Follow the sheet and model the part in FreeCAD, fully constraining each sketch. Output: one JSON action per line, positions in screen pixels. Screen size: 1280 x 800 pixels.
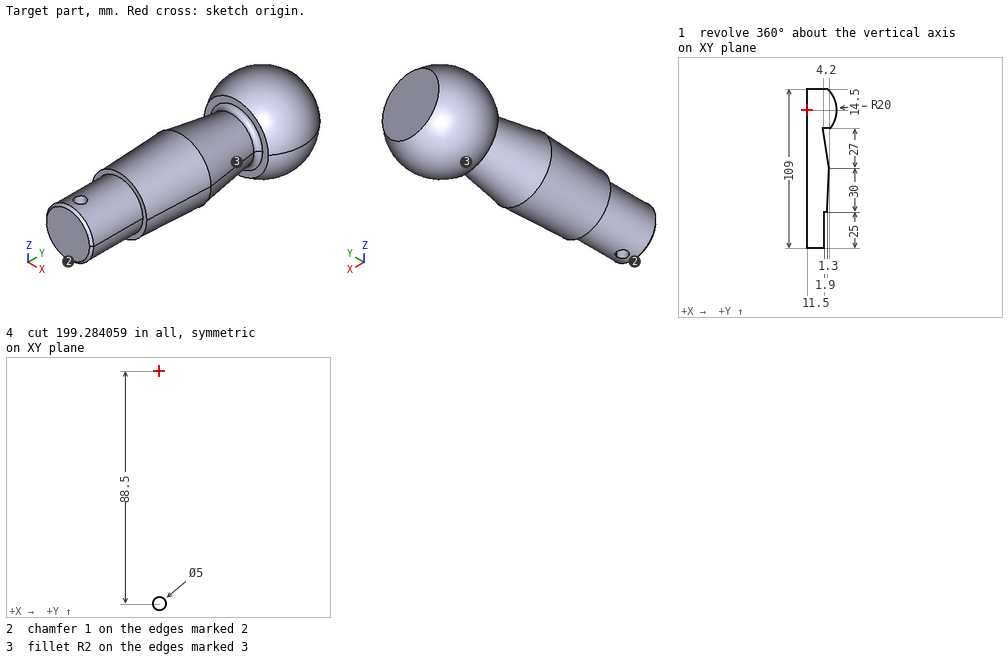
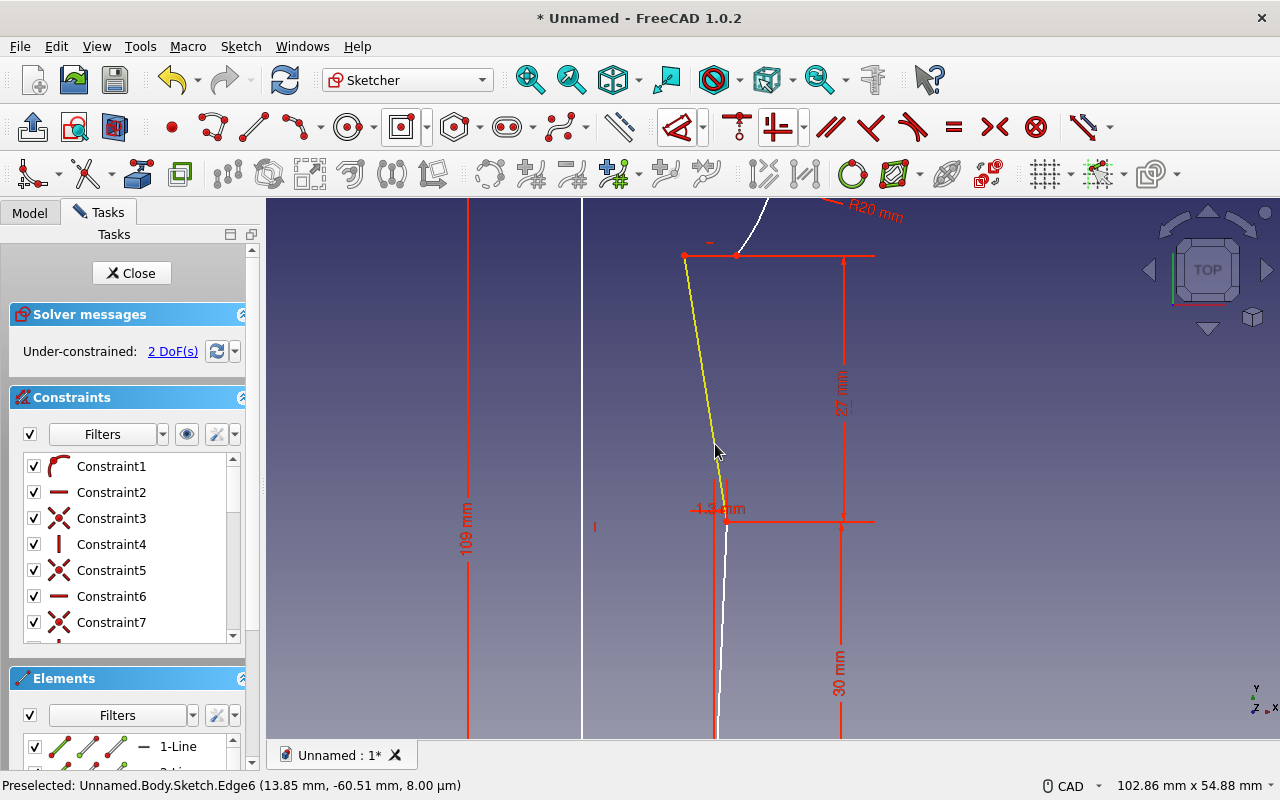
{"action": "left_click", "coordinate": [714, 442]}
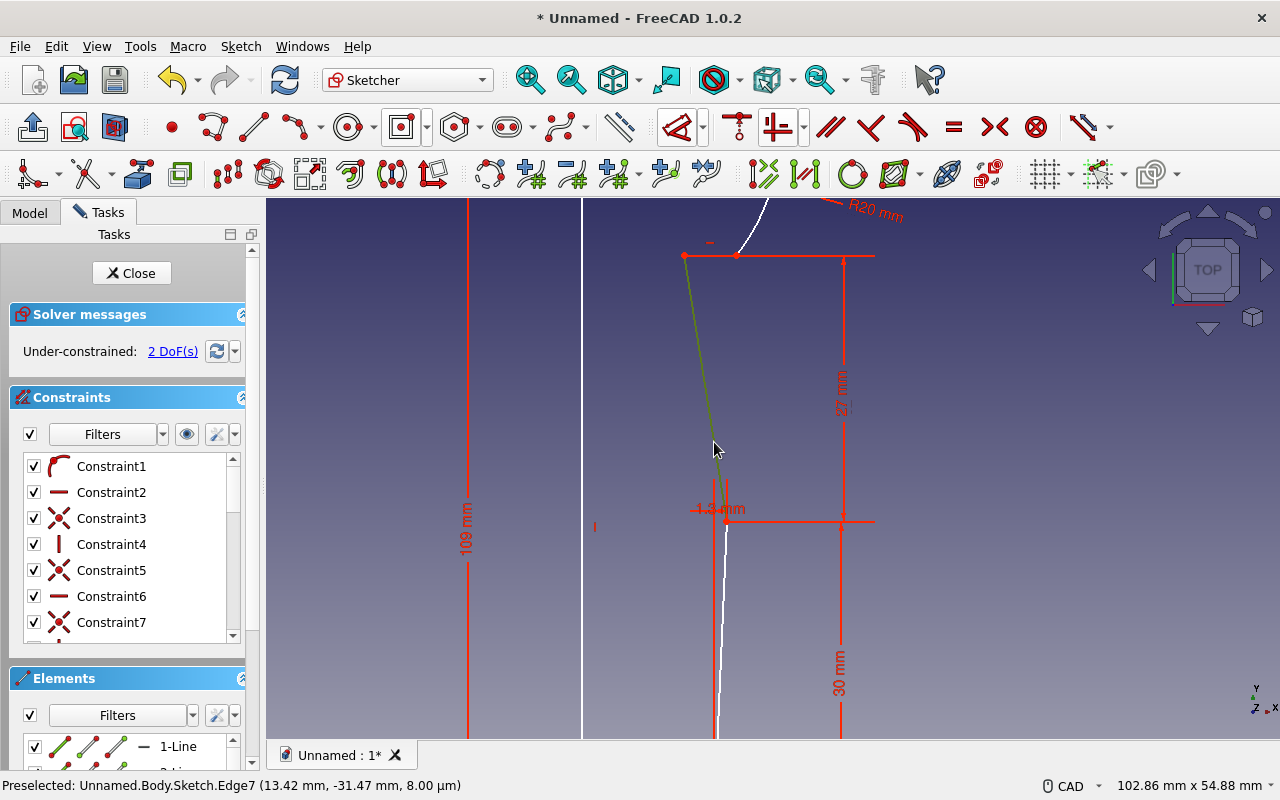
{"action": "left_click", "coordinate": [702, 128]}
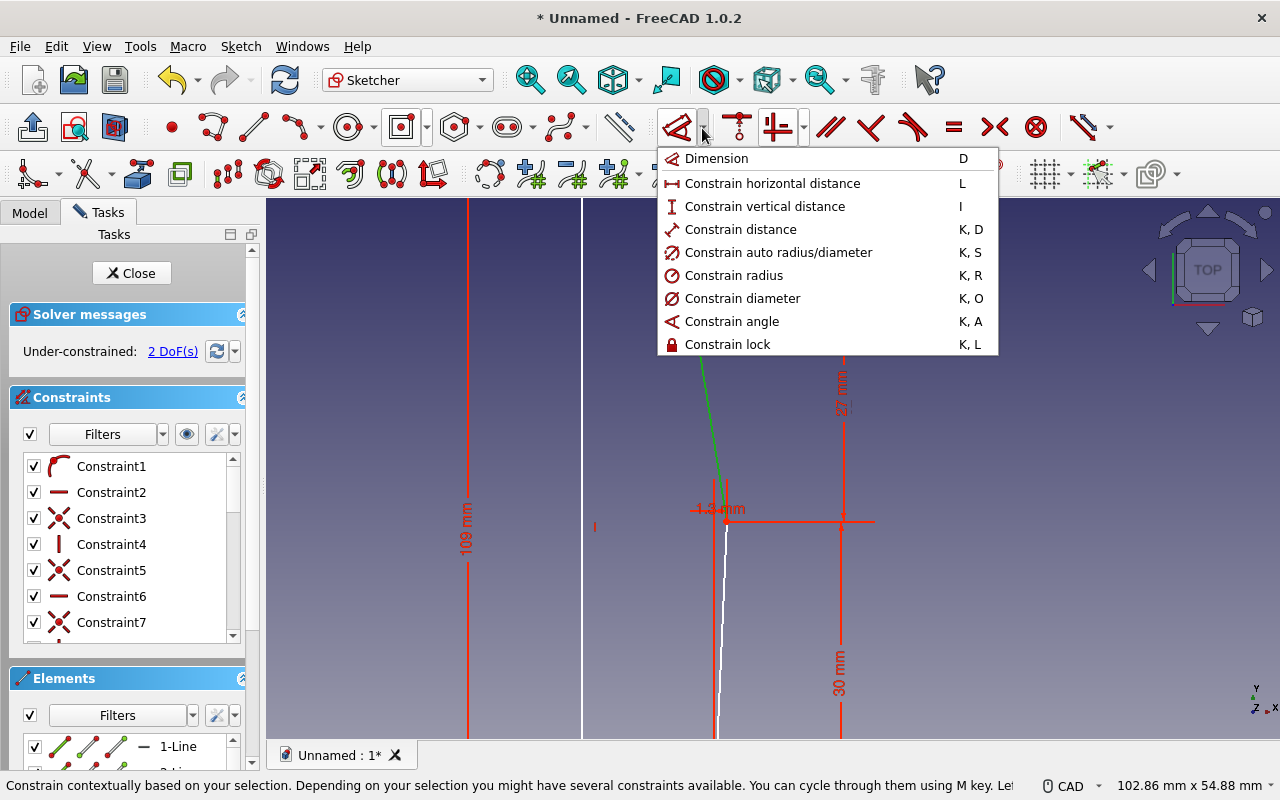
{"action": "left_click", "coordinate": [828, 184]}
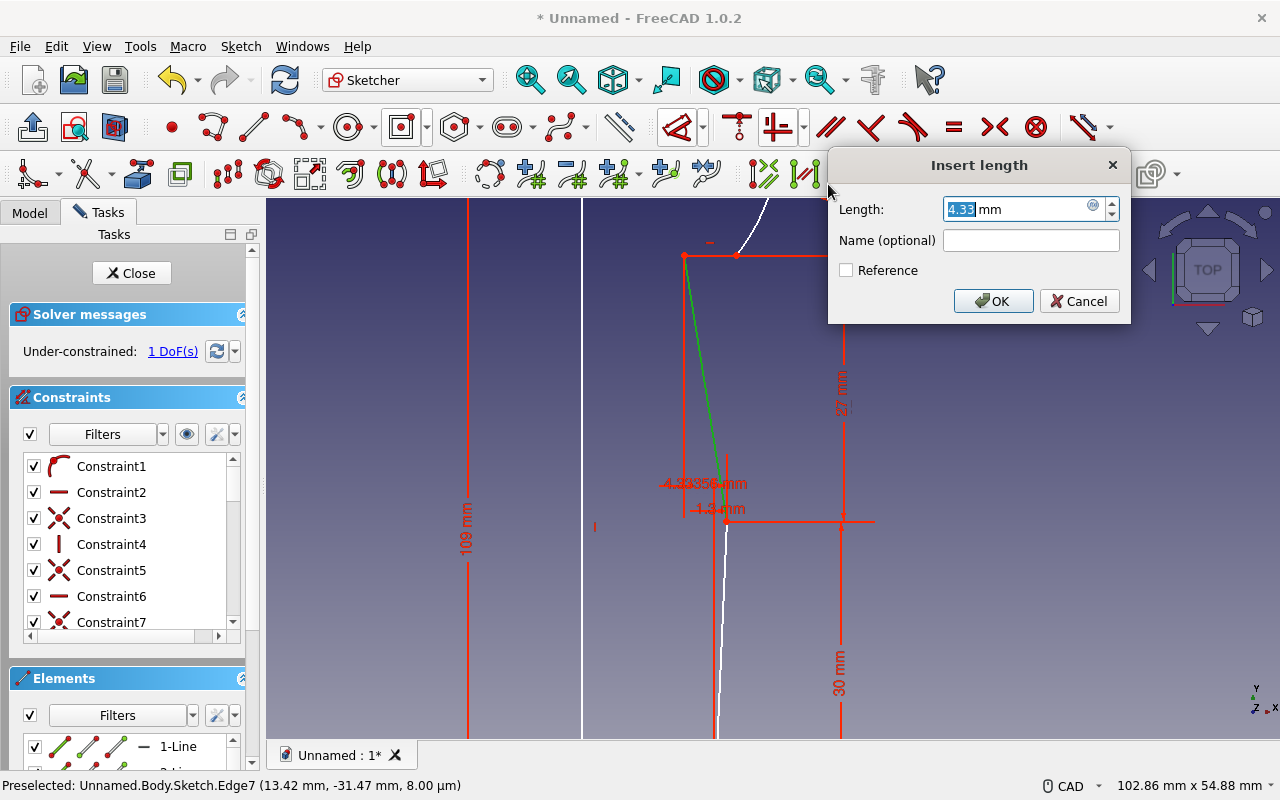
{"action": "type", "text": "4.2"}
{"action": "key", "text": "Return"}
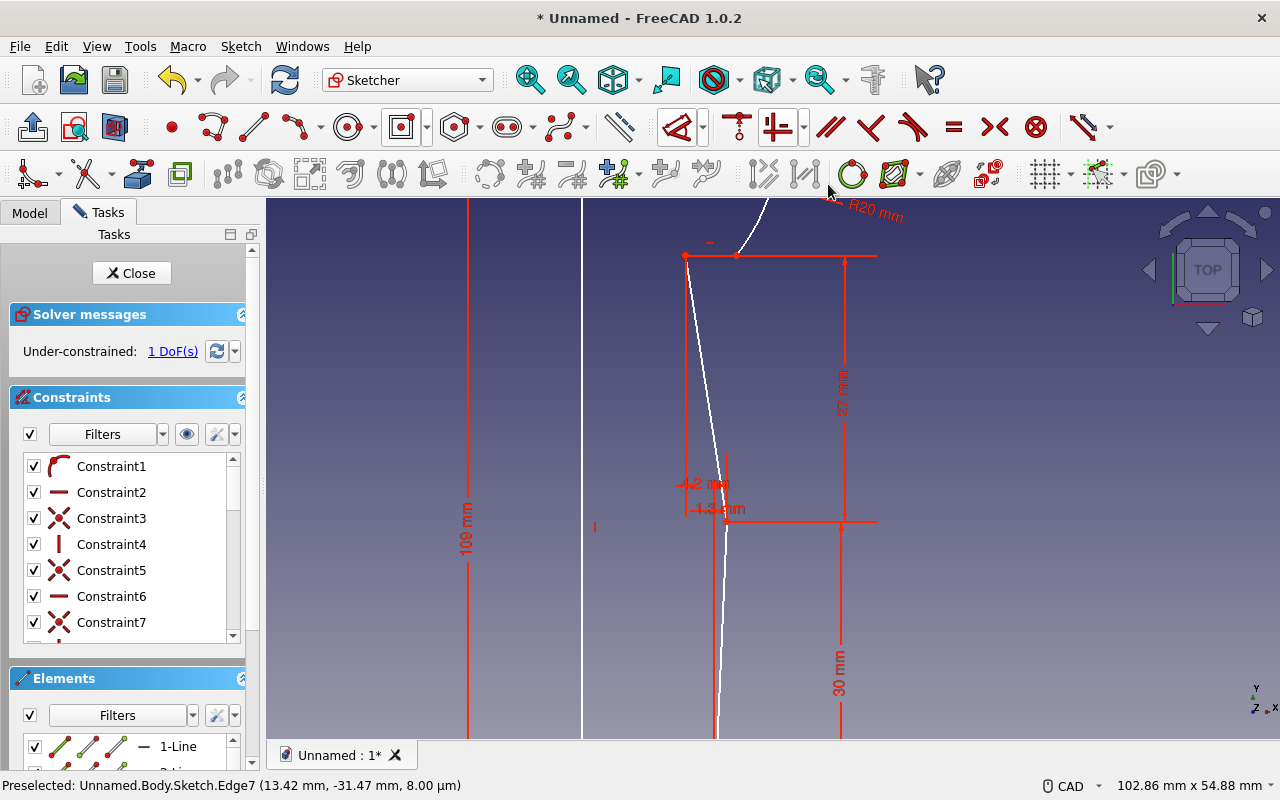
{"action": "scroll", "coordinate": [715, 443], "scroll_direction": "down", "scroll_amount": 6}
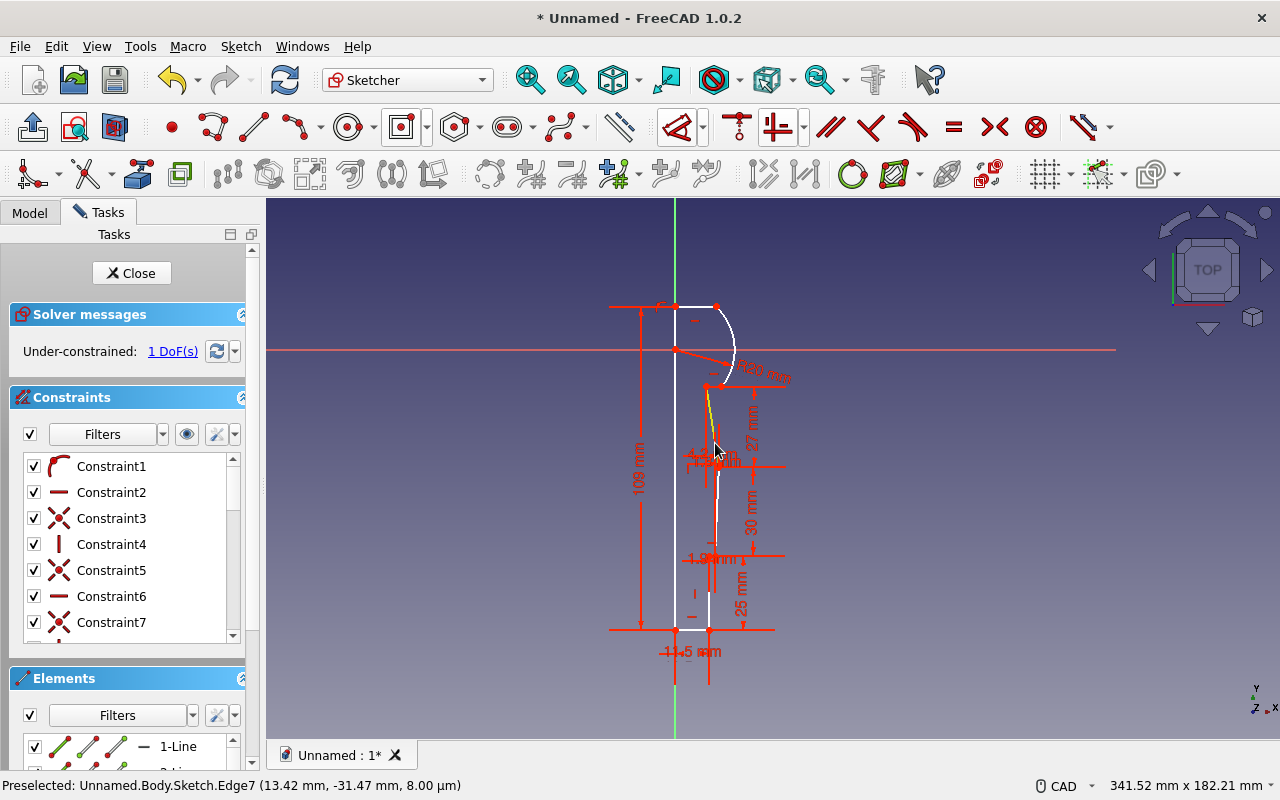
{"action": "left_click", "coordinate": [716, 307]}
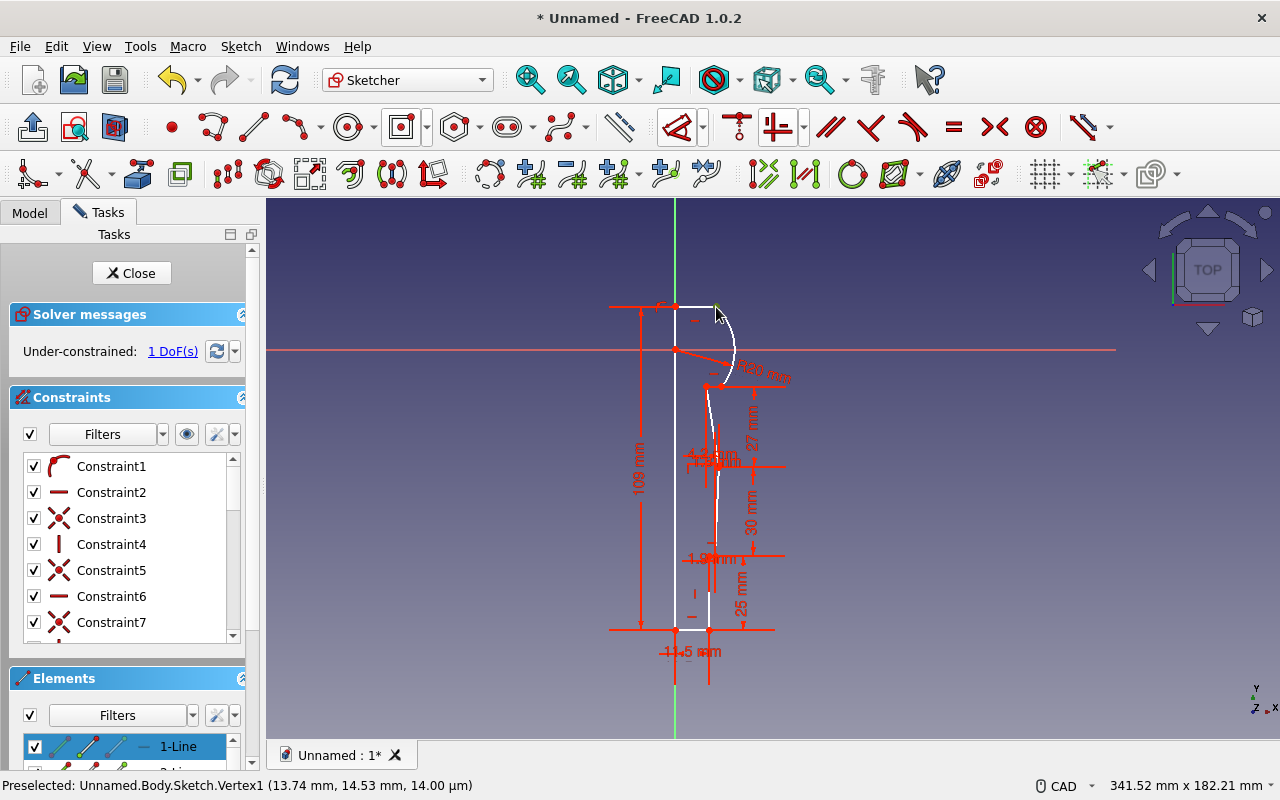
{"action": "key", "text": "i"}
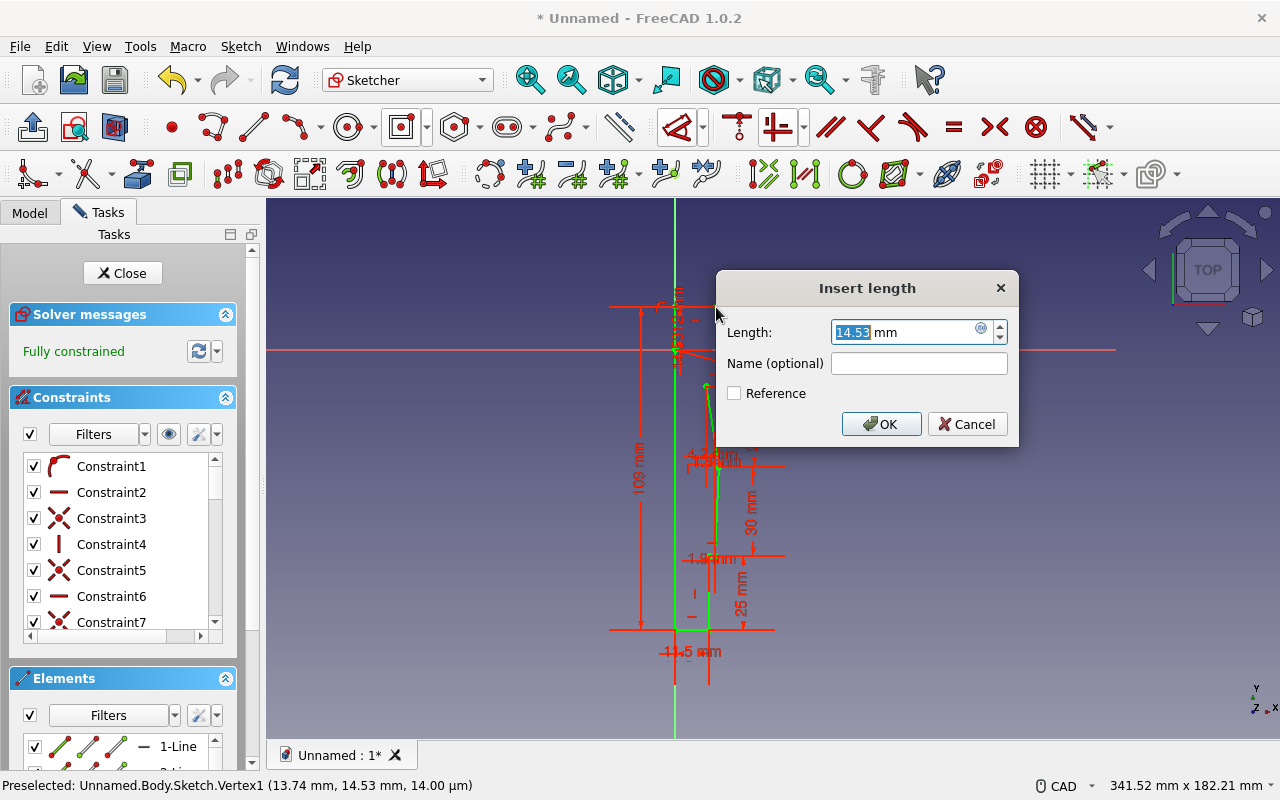
{"action": "type", "text": "14.5"}
{"action": "key", "text": "Return"}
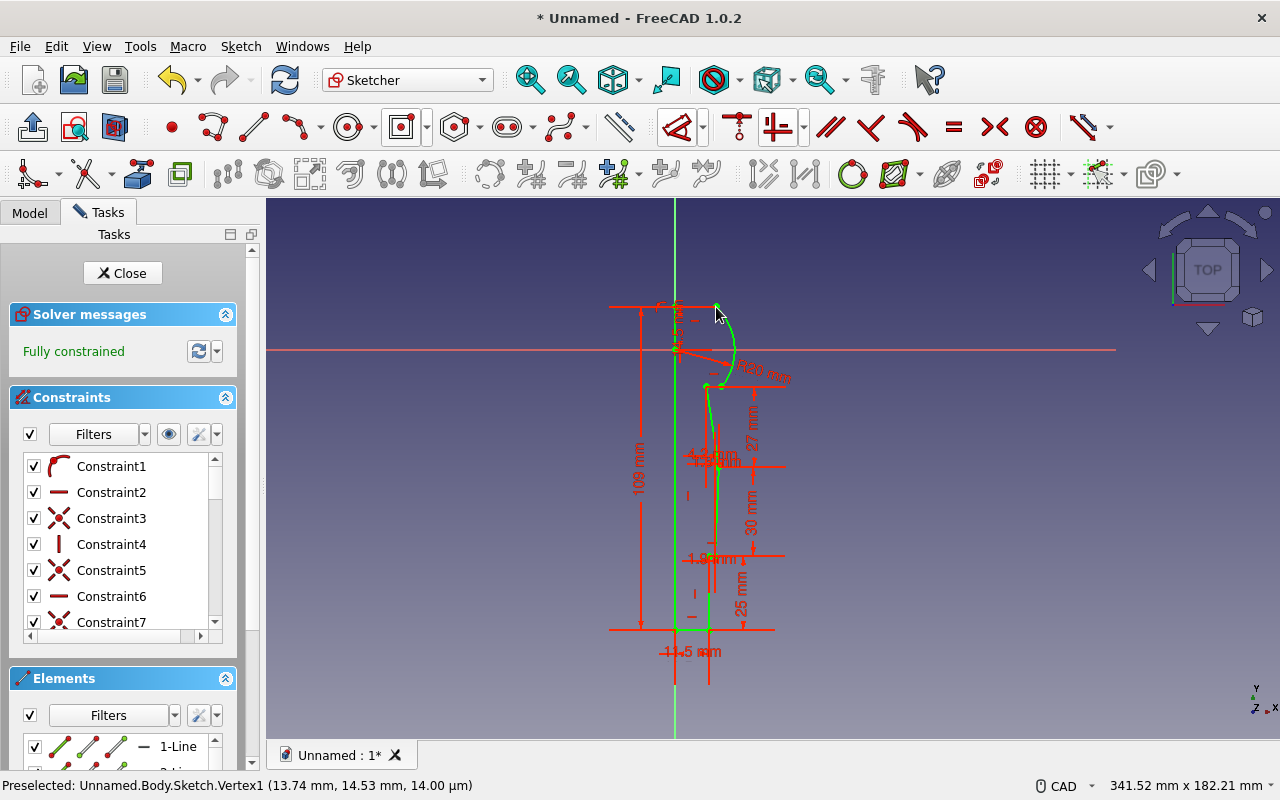
{"action": "left_click", "coordinate": [123, 273]}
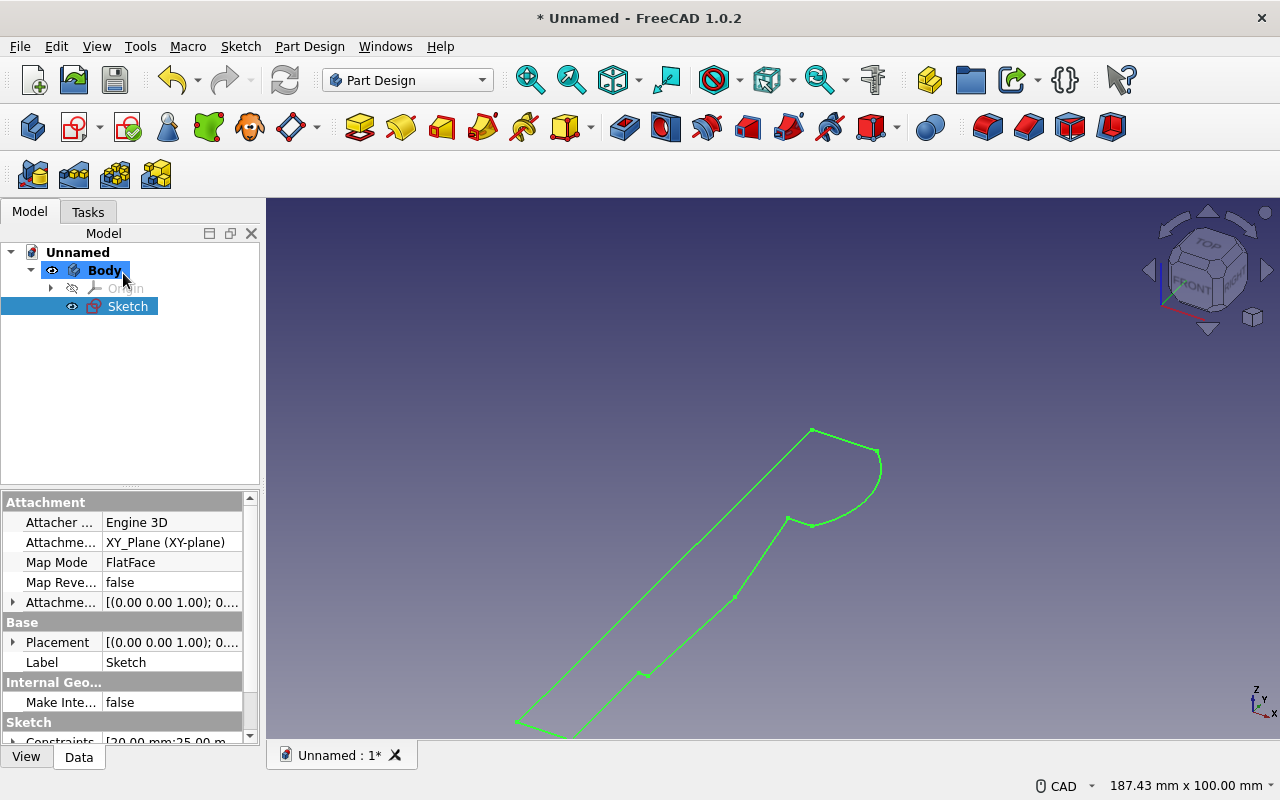
{"action": "left_click", "coordinate": [401, 128]}